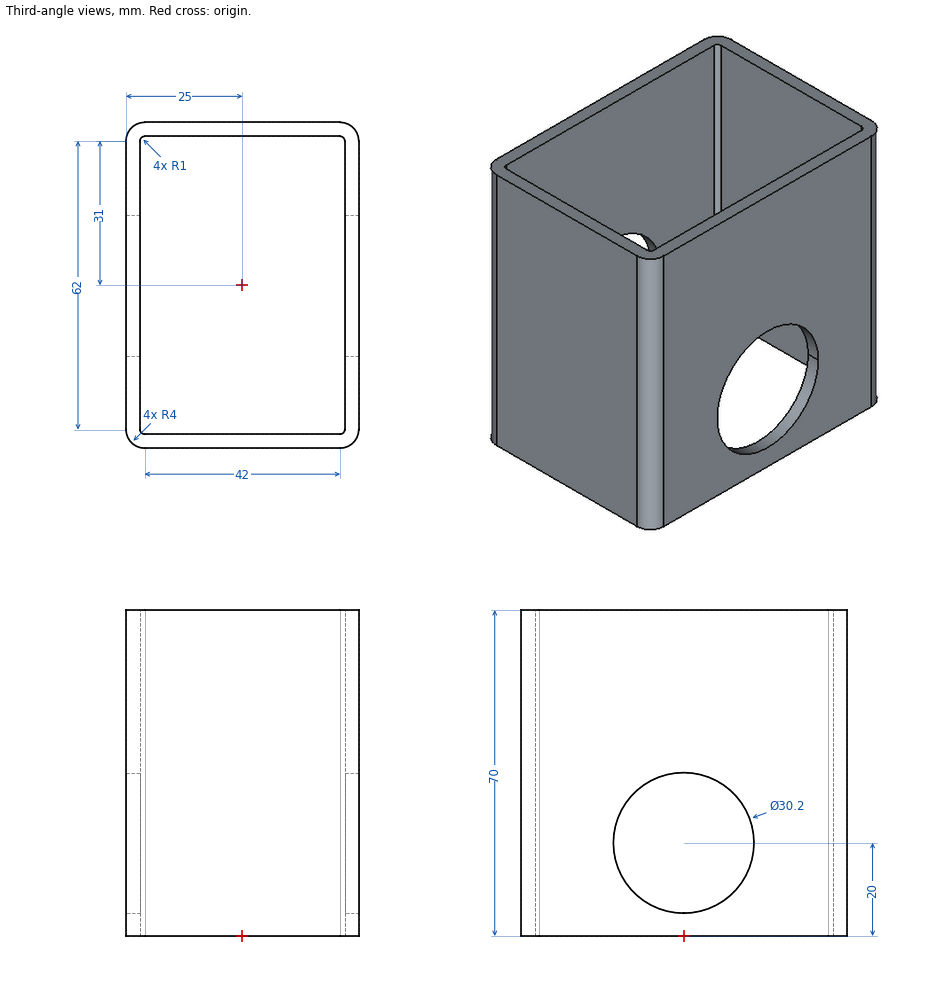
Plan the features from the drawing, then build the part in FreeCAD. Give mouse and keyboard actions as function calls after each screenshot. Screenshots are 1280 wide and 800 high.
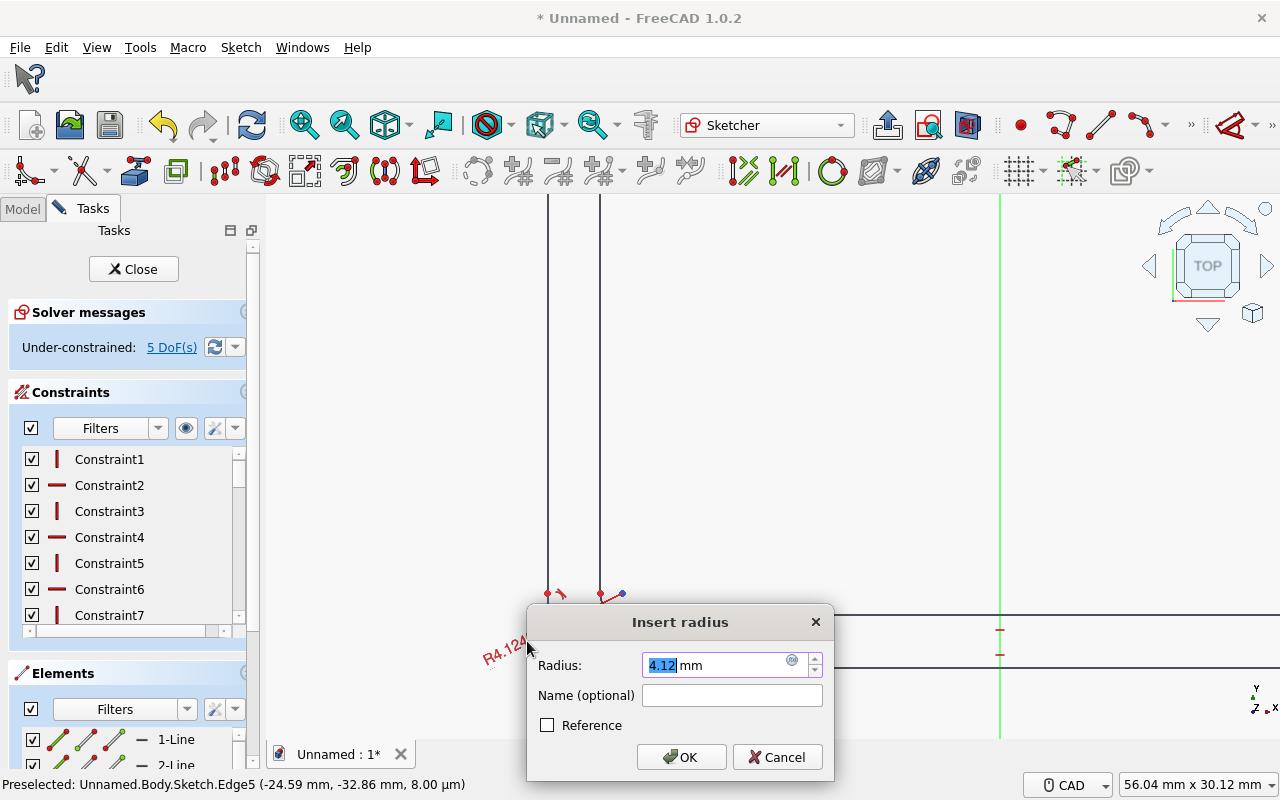
text(4)
key(Return)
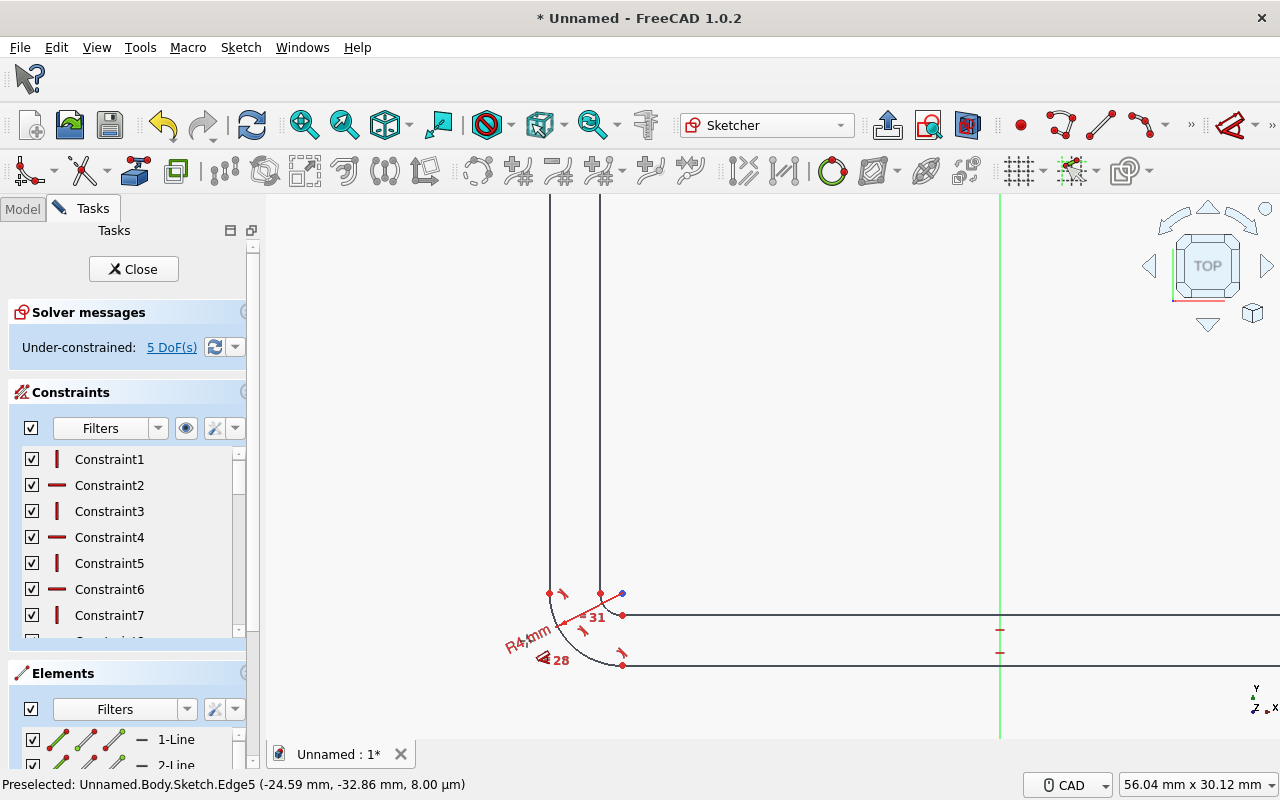
scroll(608, 609, down, 7)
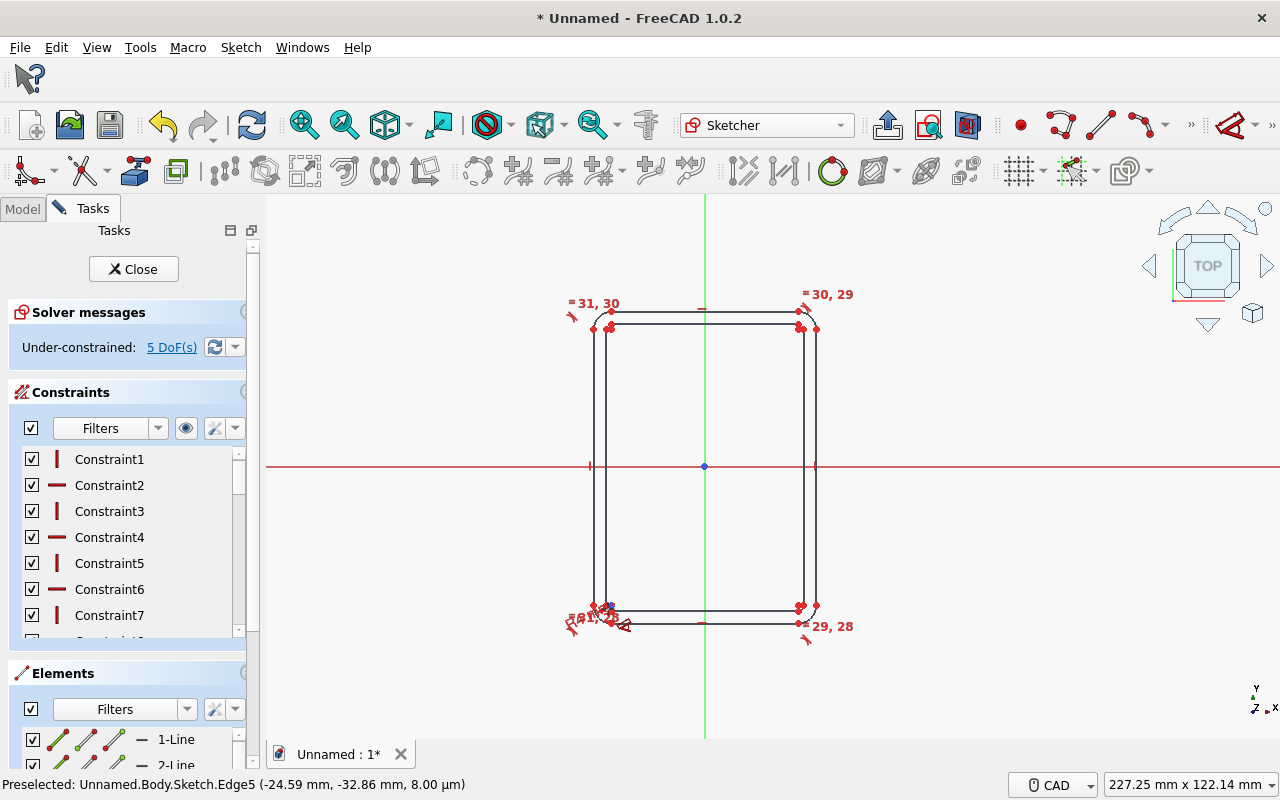
scroll(609, 325, up, 11)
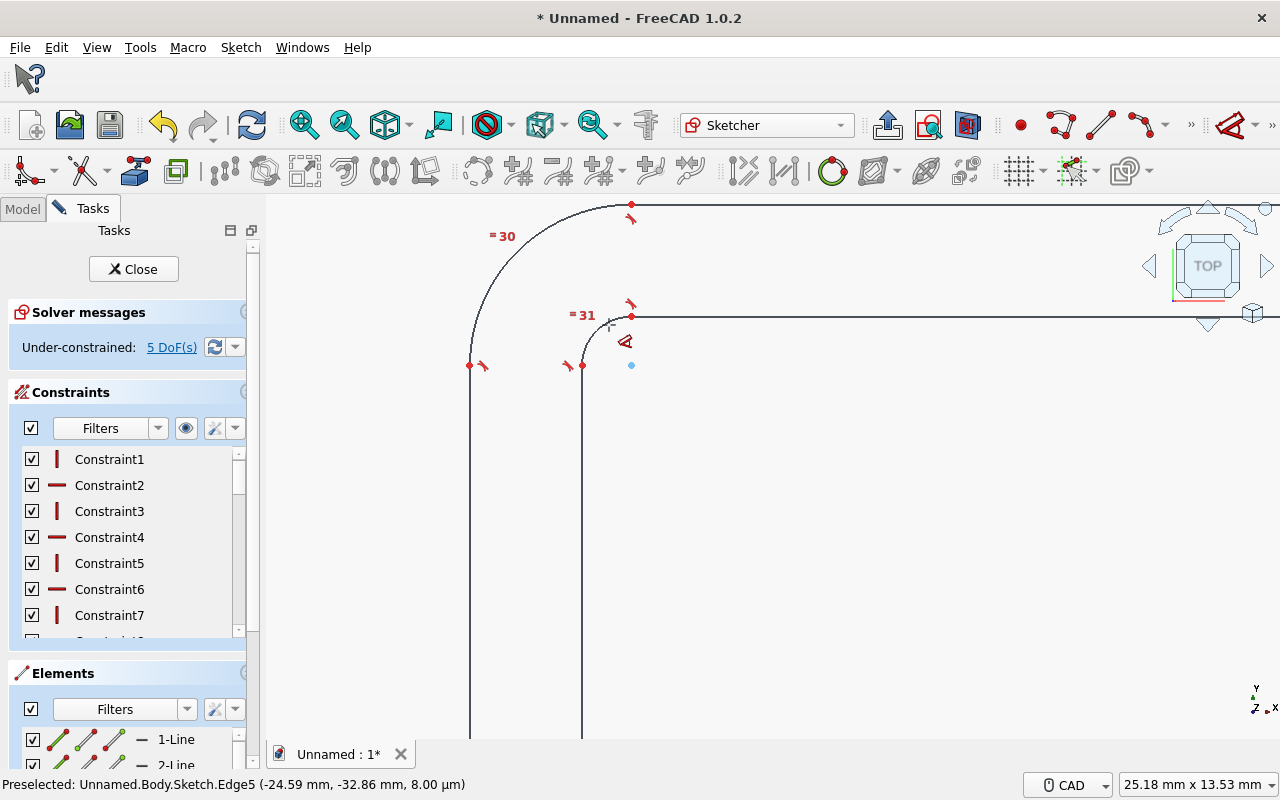
click(609, 322)
click(595, 293)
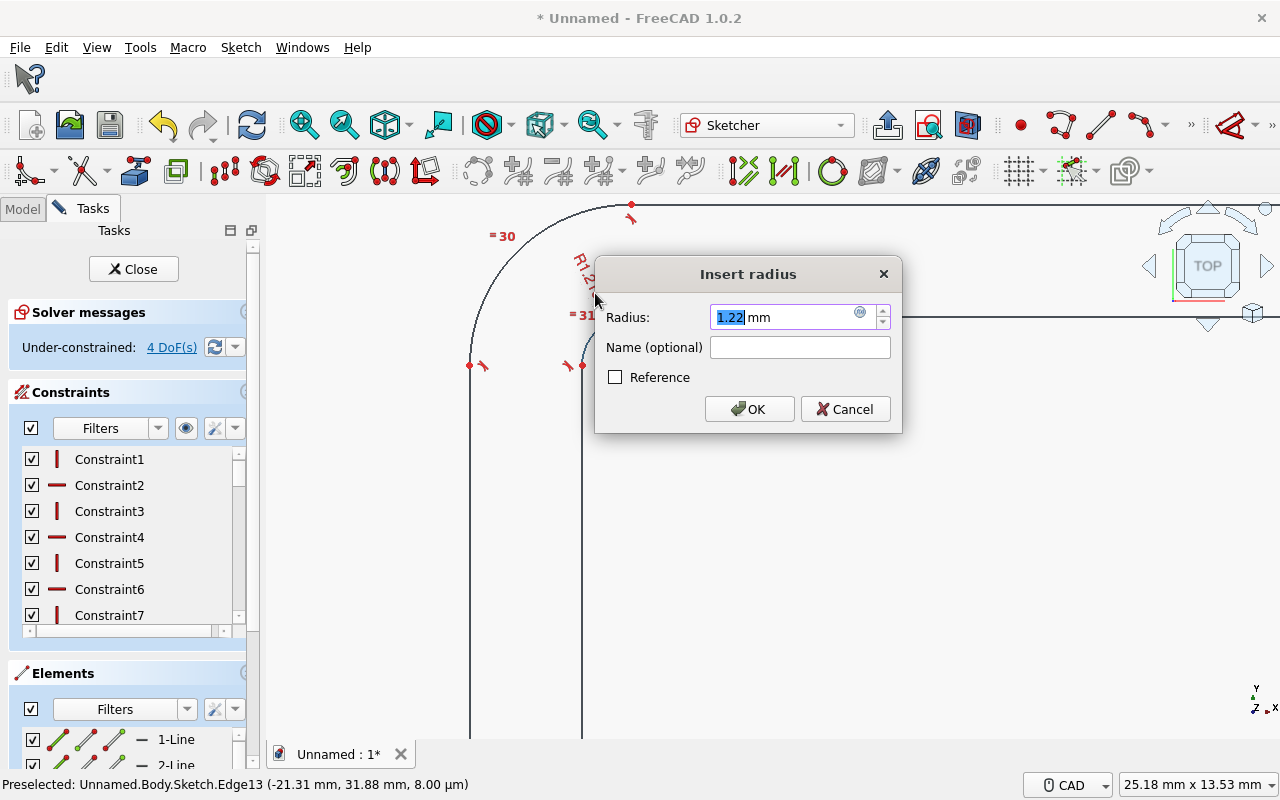
text(1)
key(Return)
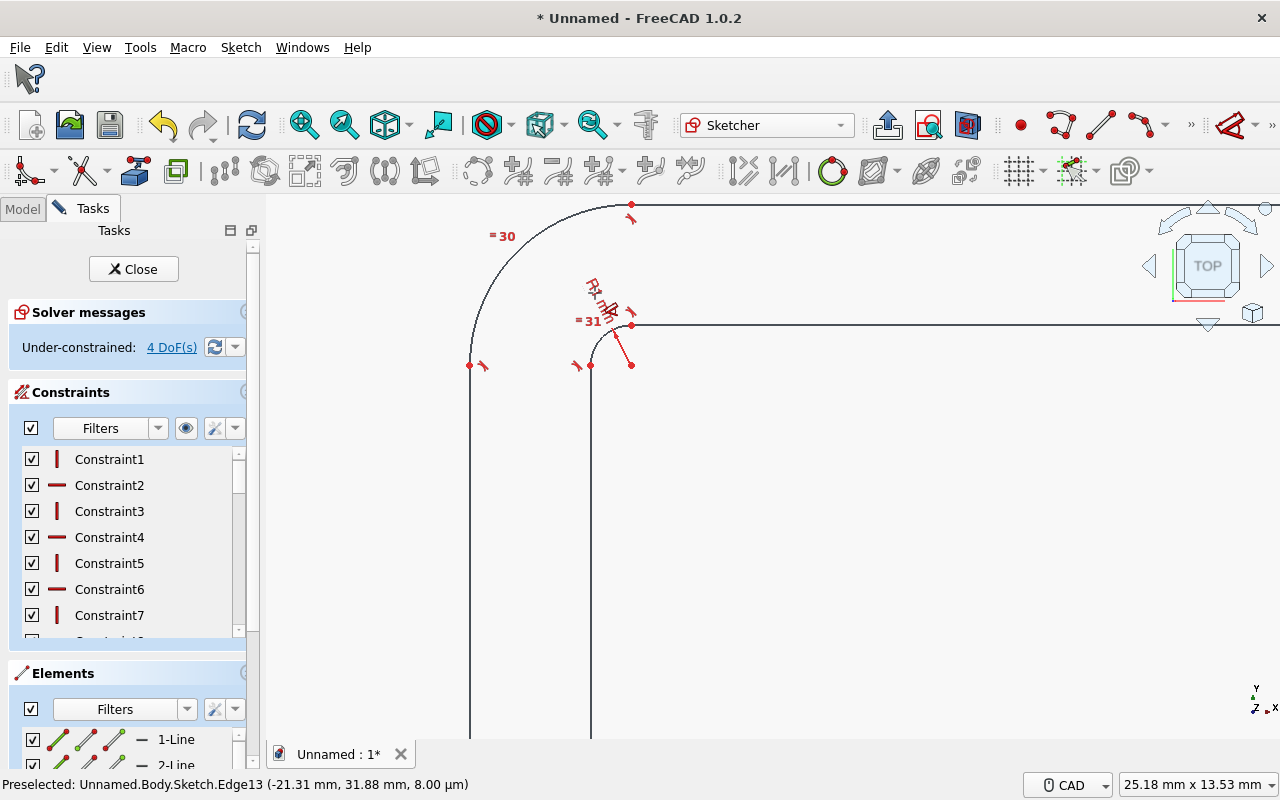
scroll(609, 325, down, 11)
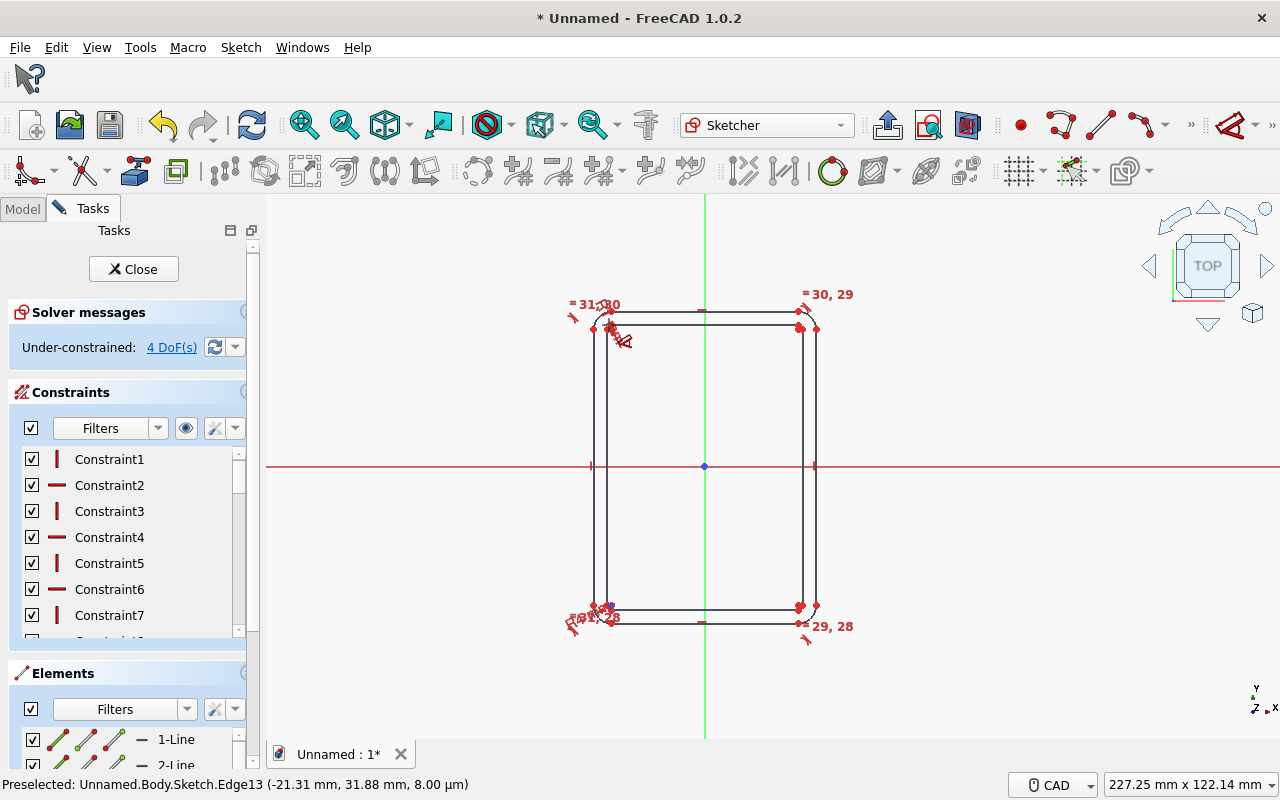
click(594, 413)
click(560, 404)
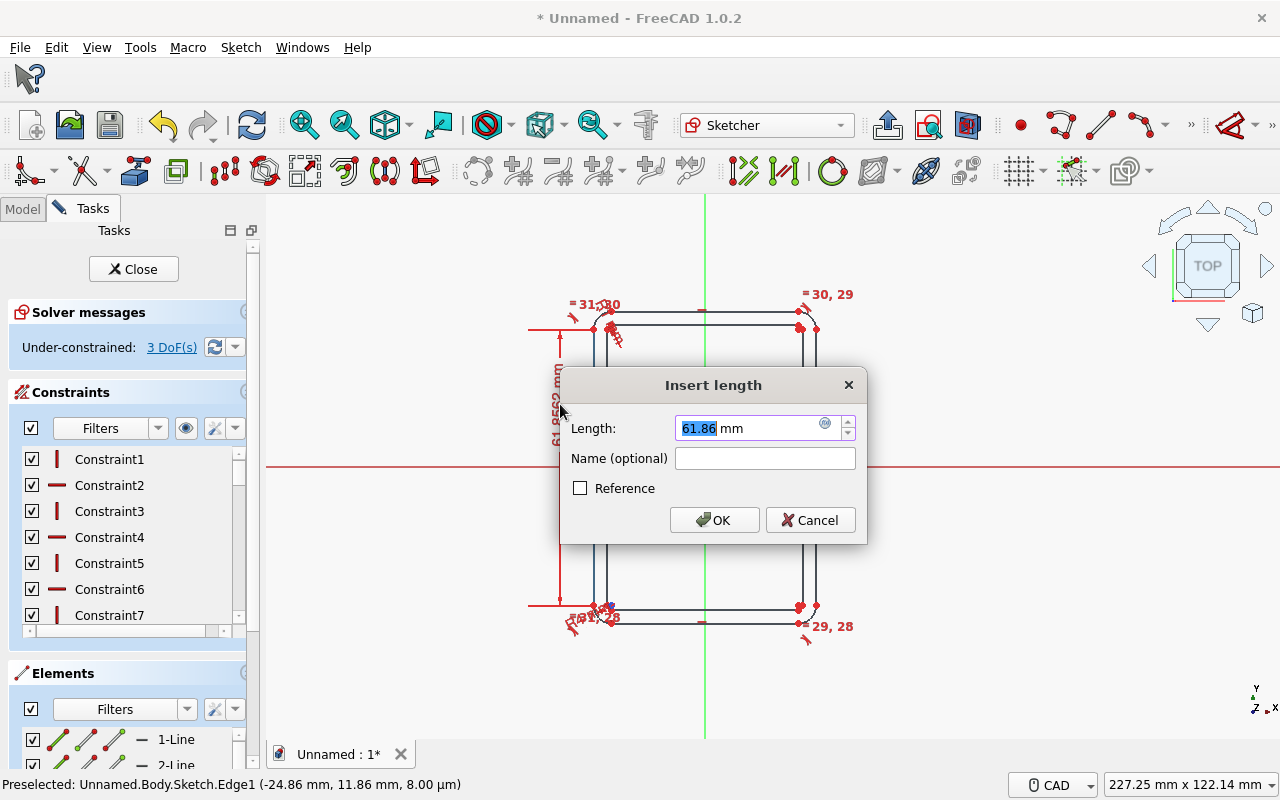
text(62)
key(Return)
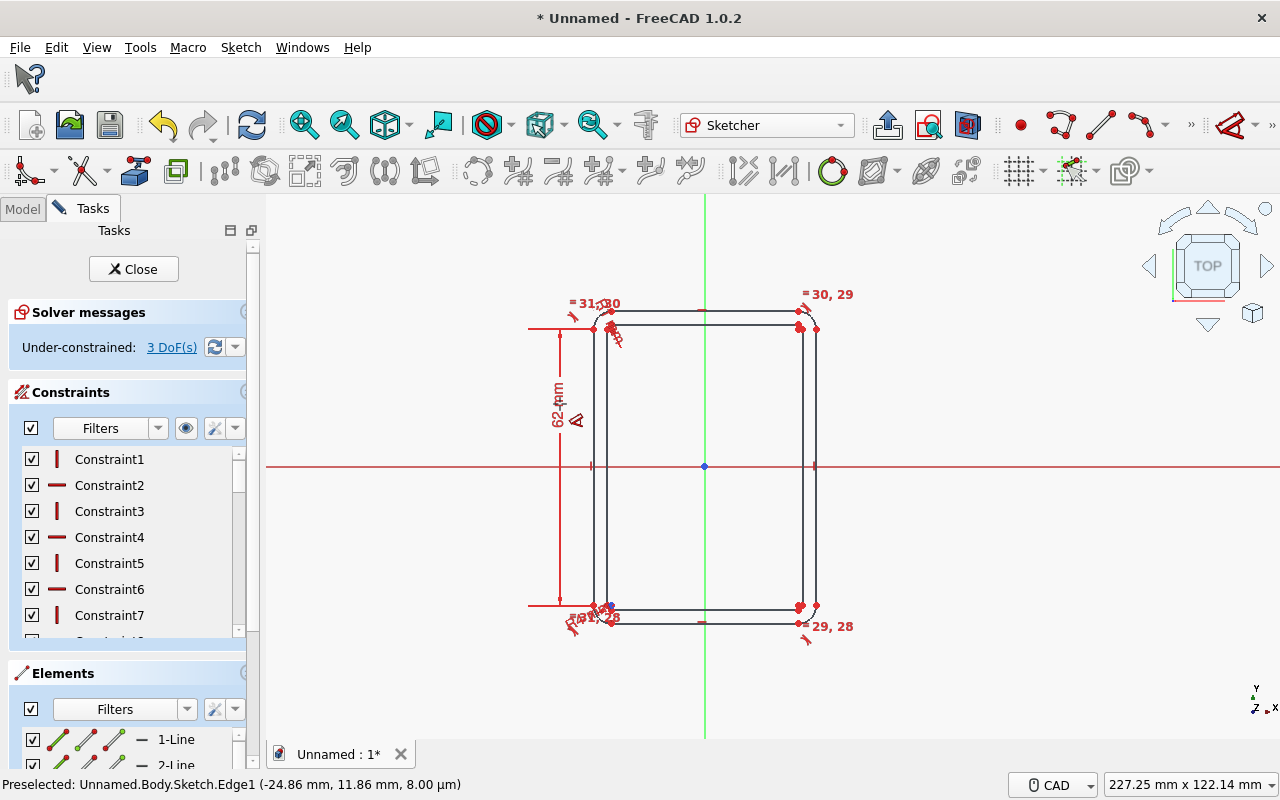
click(668, 624)
click(662, 658)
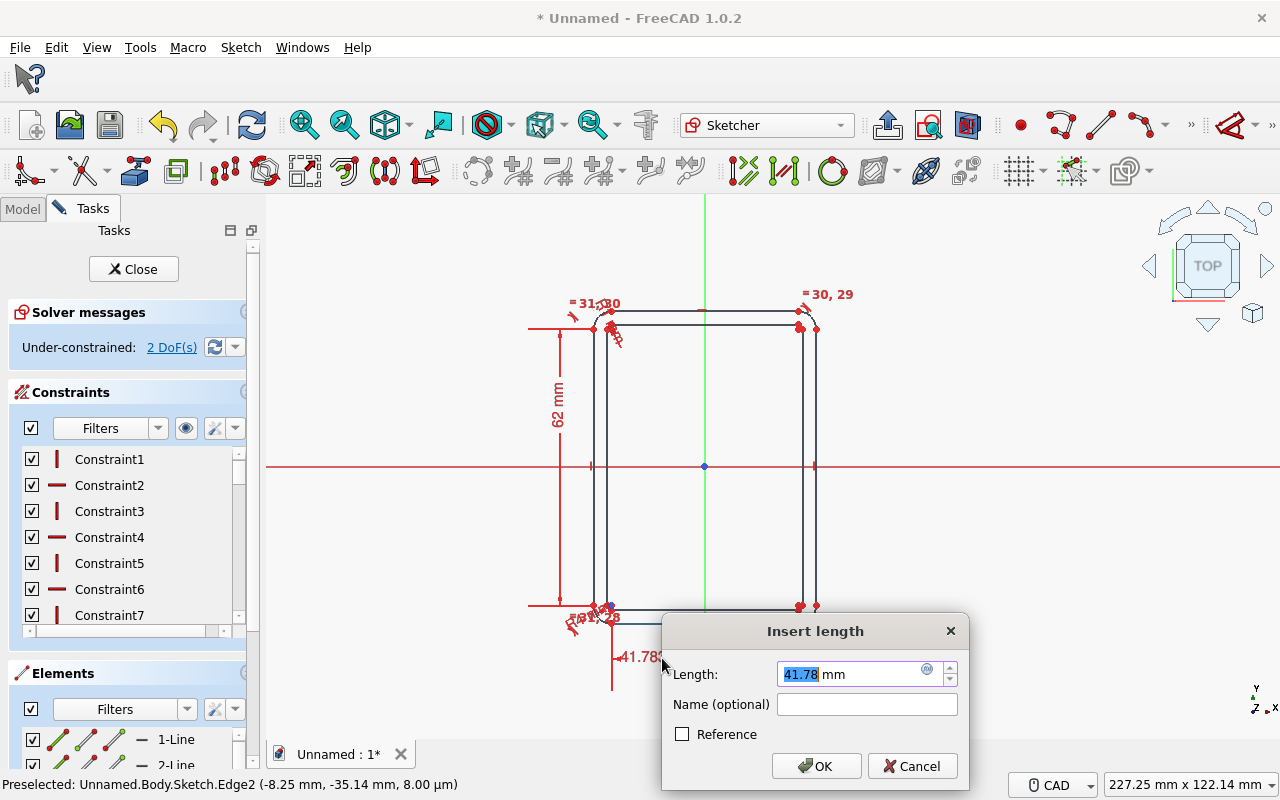
text(42)
key(Return)